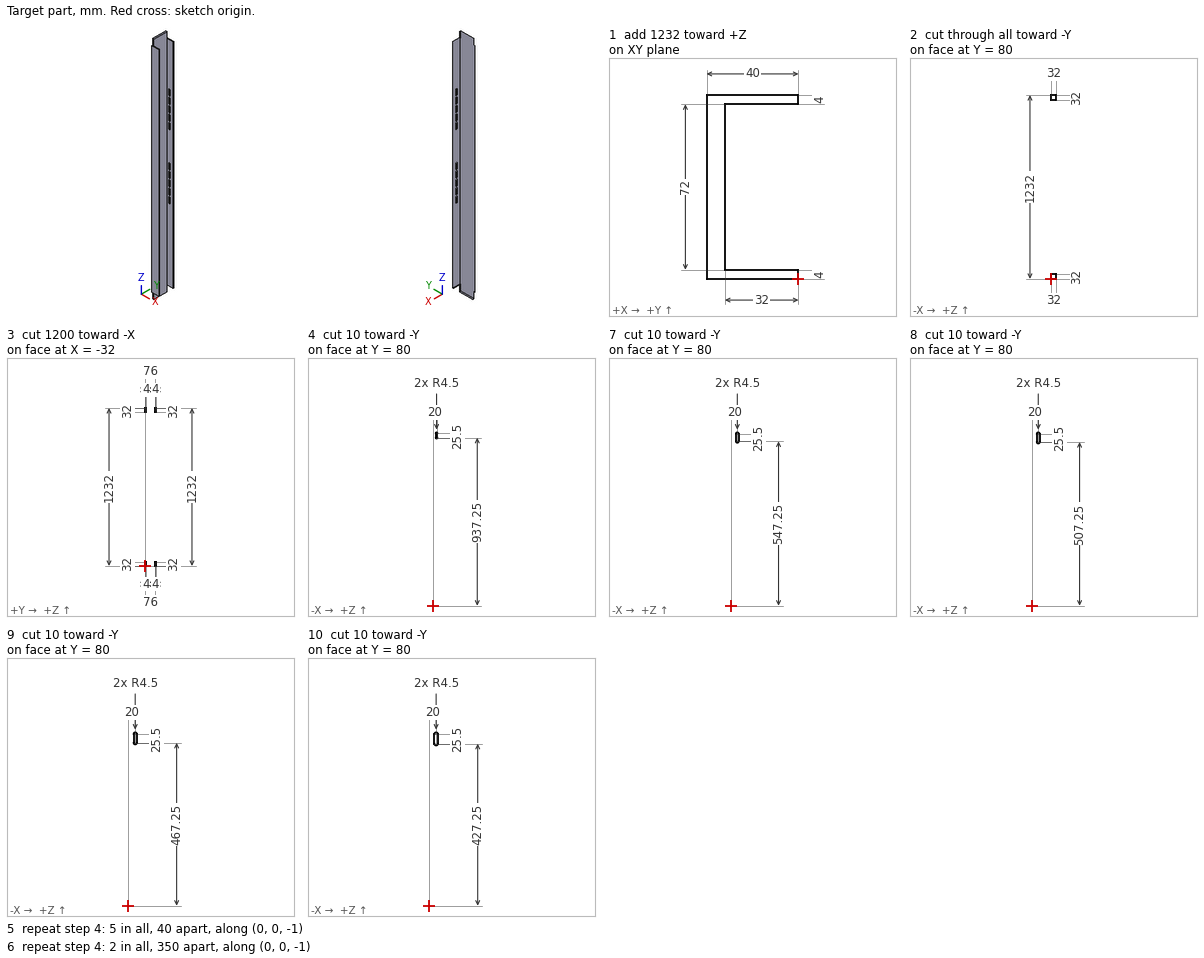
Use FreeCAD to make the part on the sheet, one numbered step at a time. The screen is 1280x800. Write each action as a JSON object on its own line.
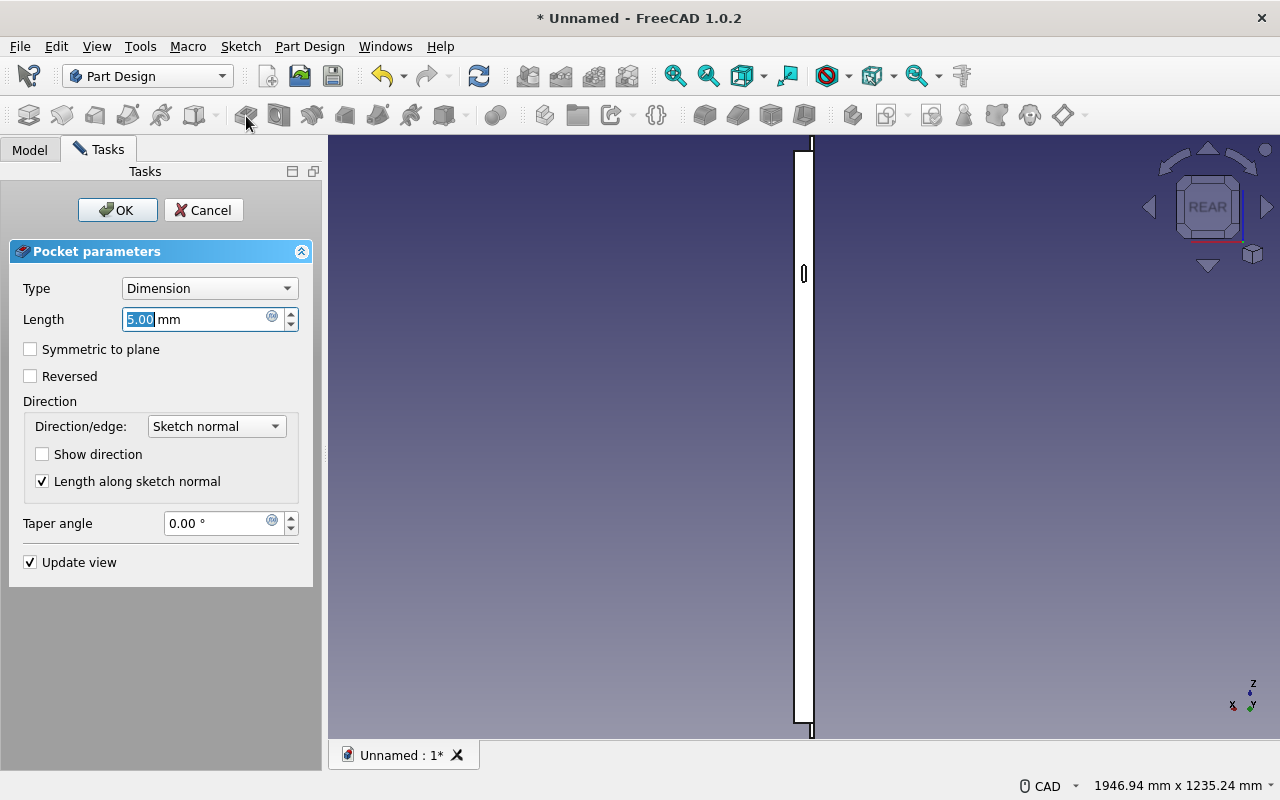
{"action": "type", "text": "10"}
{"action": "key", "text": "Tab"}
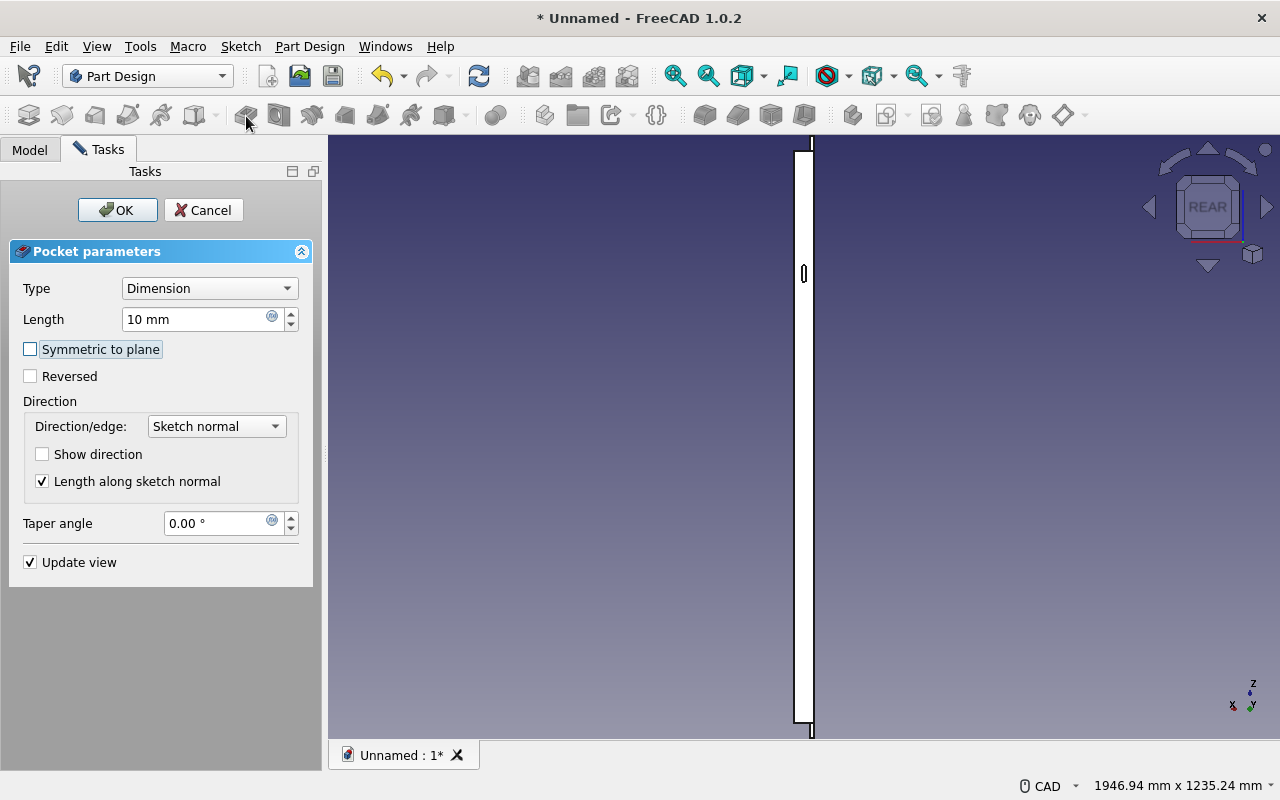
{"action": "left_click", "coordinate": [118, 210]}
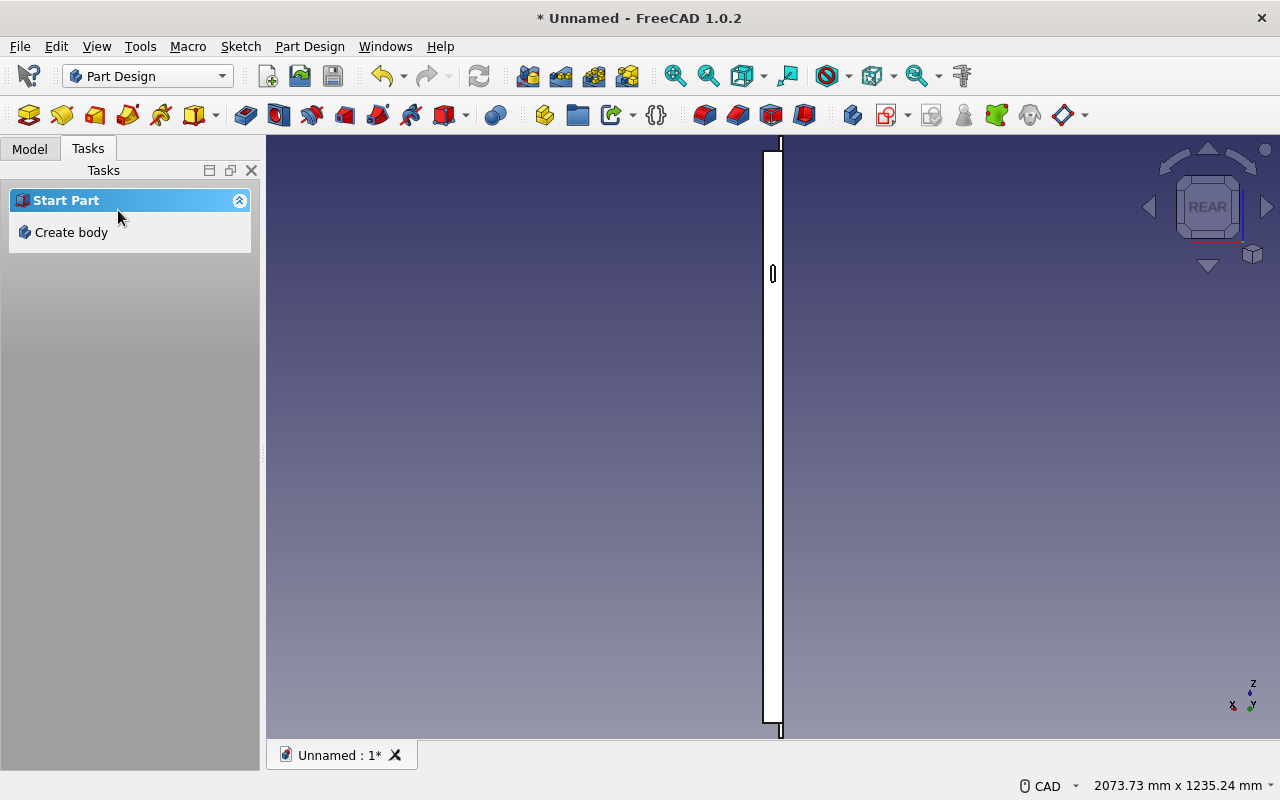
{"action": "left_click", "coordinate": [30, 148]}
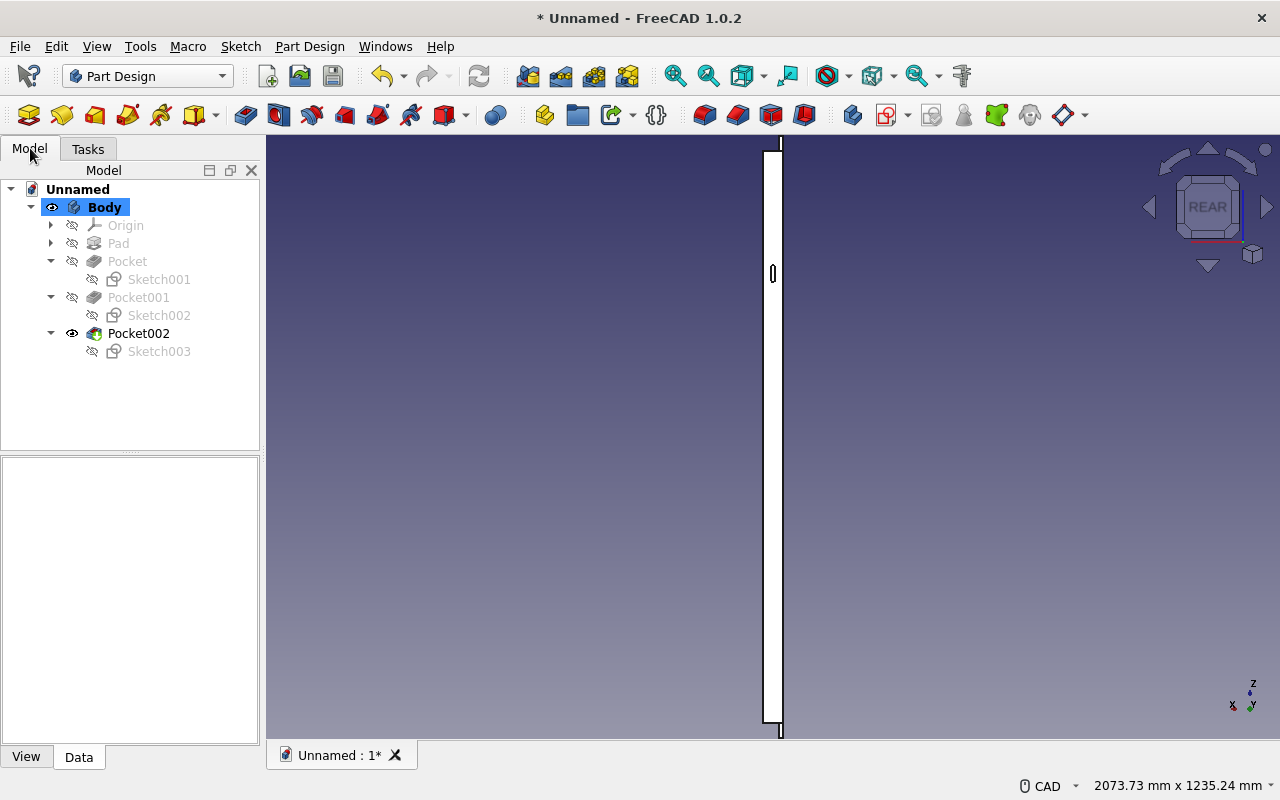
{"action": "left_click", "coordinate": [117, 333]}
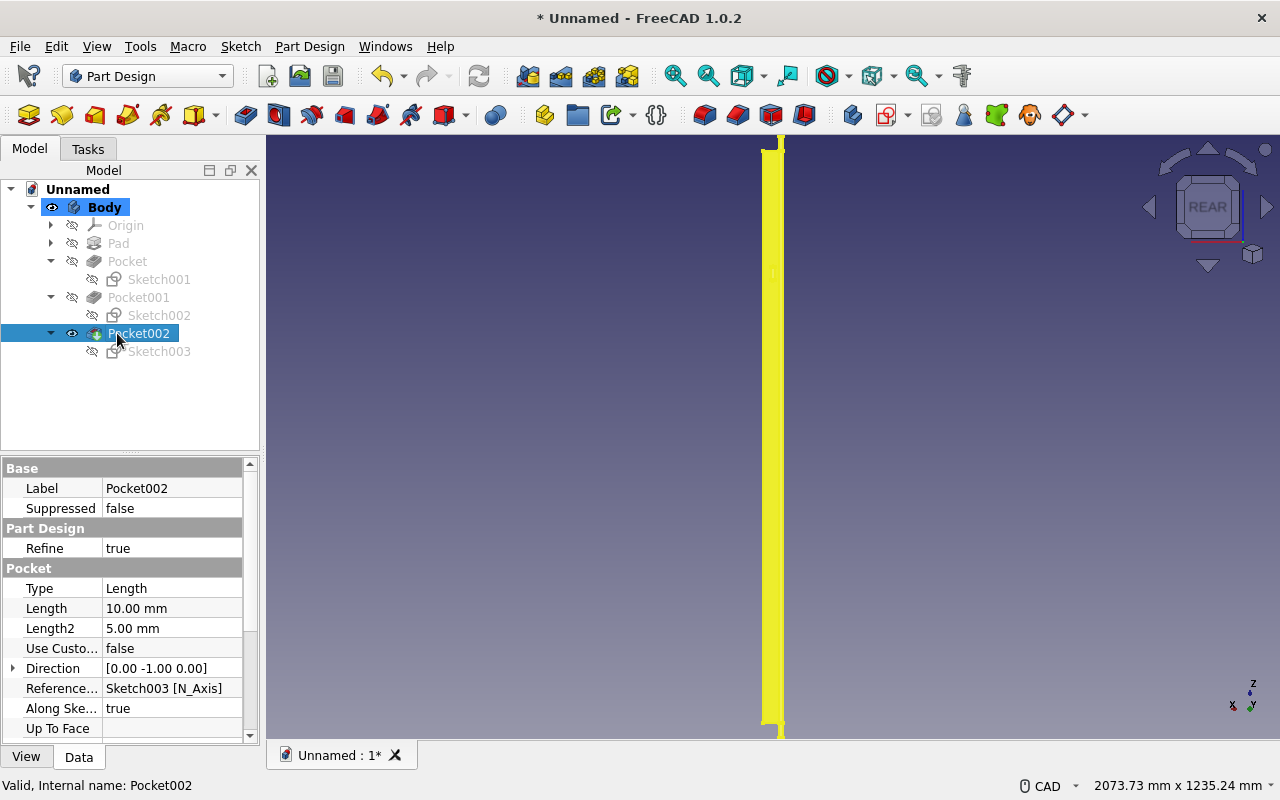
{"action": "left_click", "coordinate": [561, 76]}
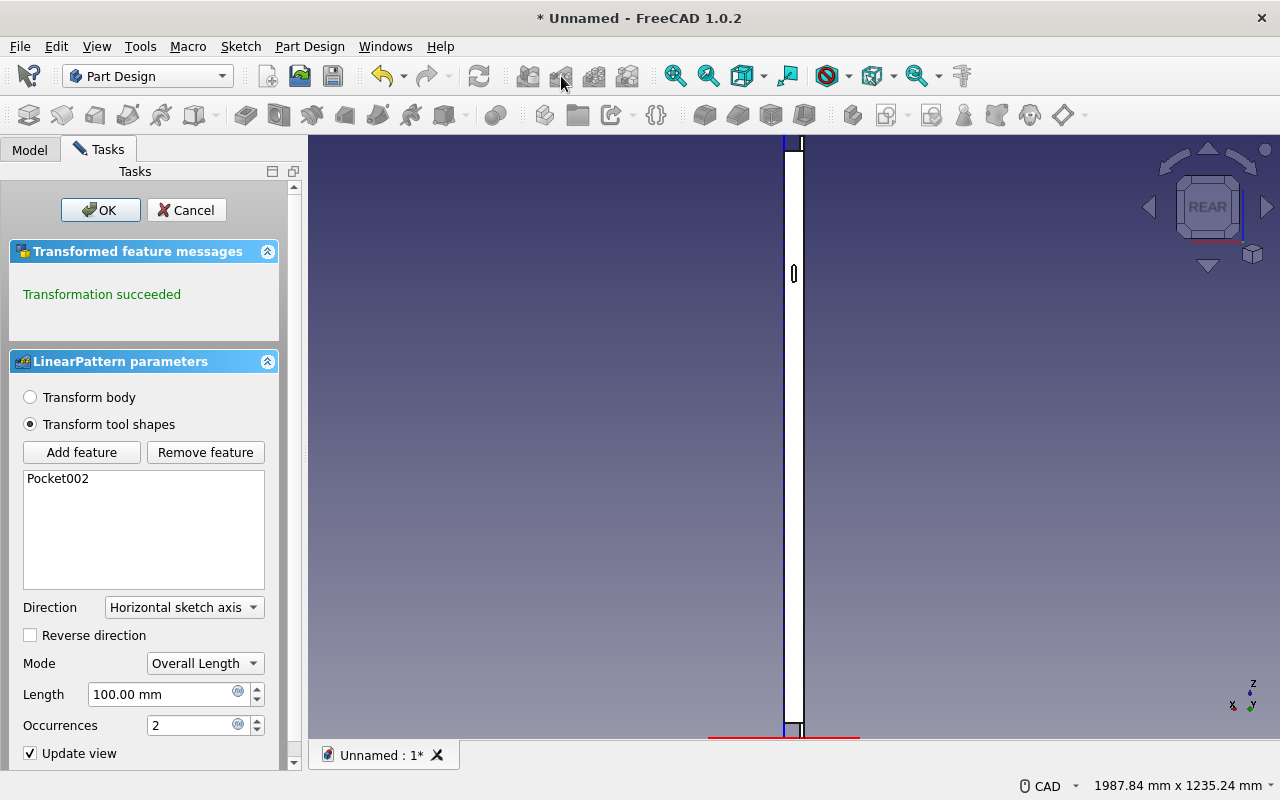
{"action": "left_click", "coordinate": [185, 608]}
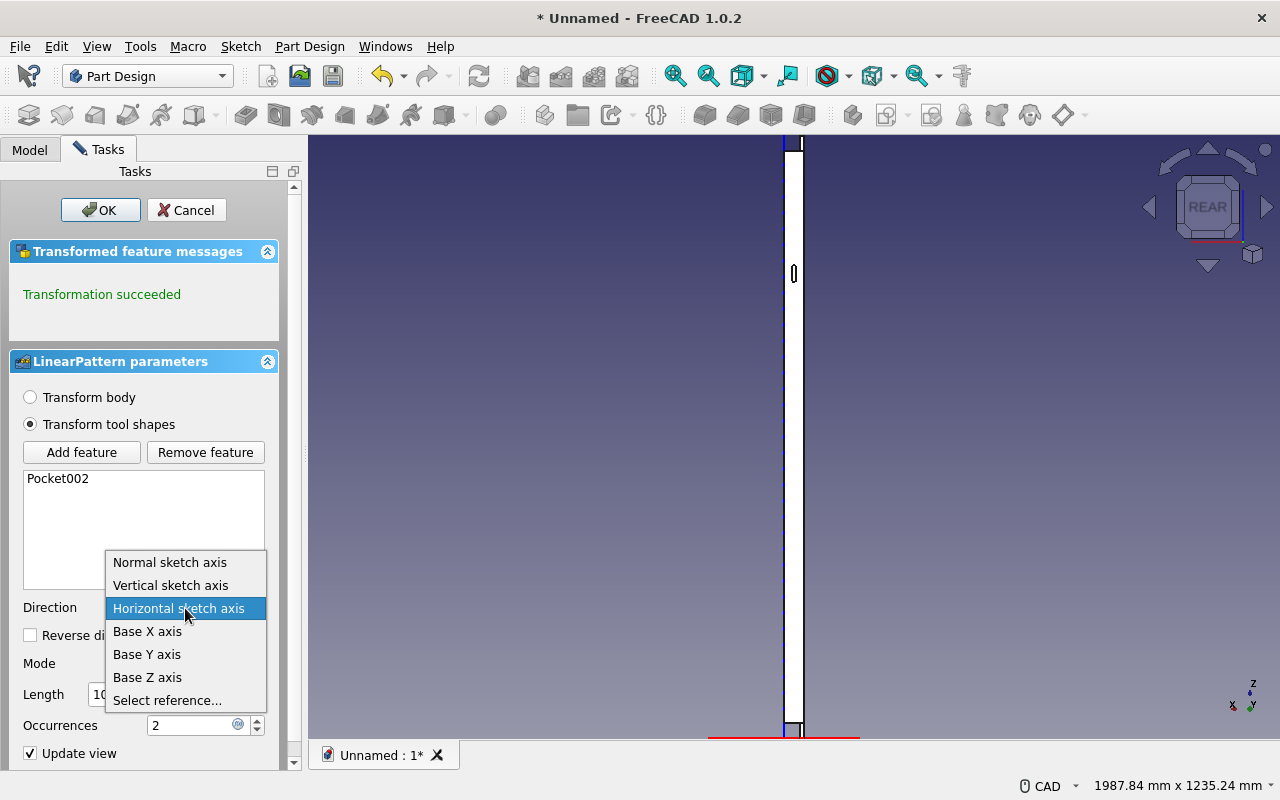
{"action": "left_click", "coordinate": [184, 678]}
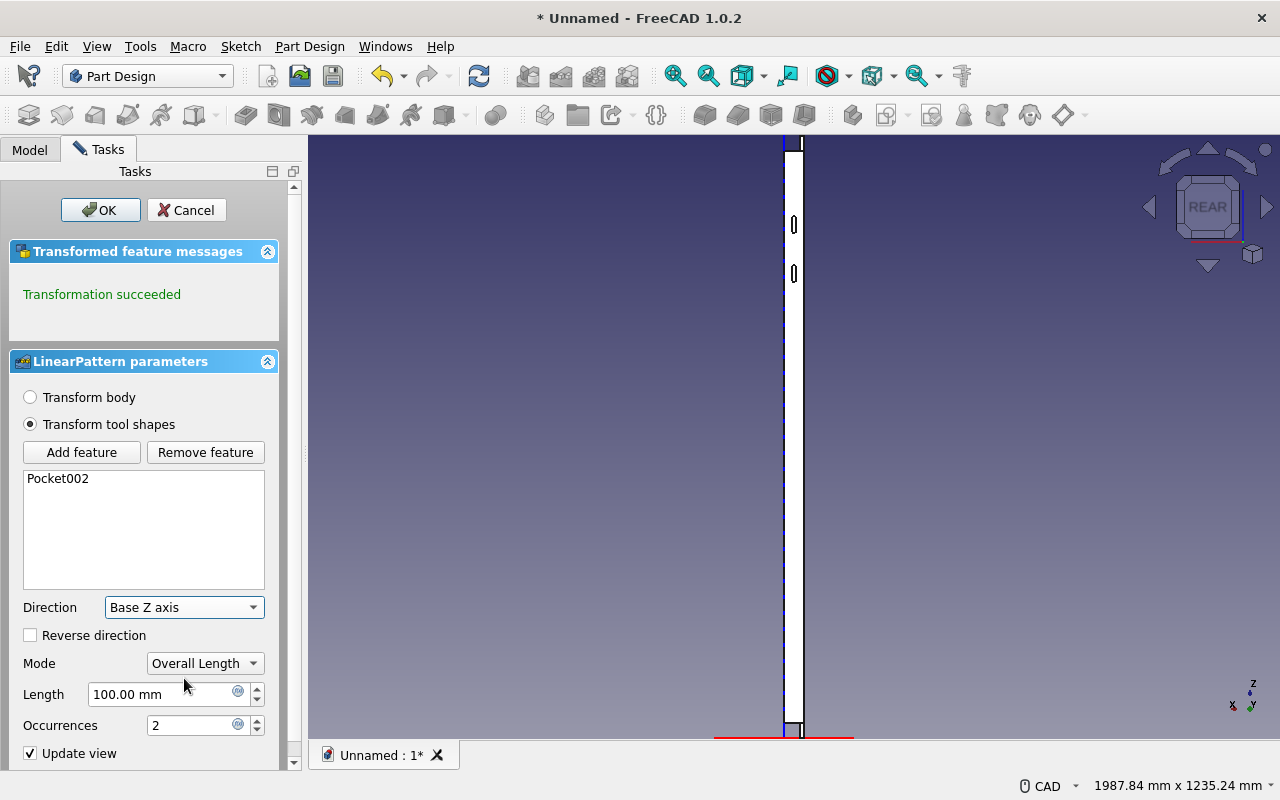
{"action": "left_click", "coordinate": [206, 664]}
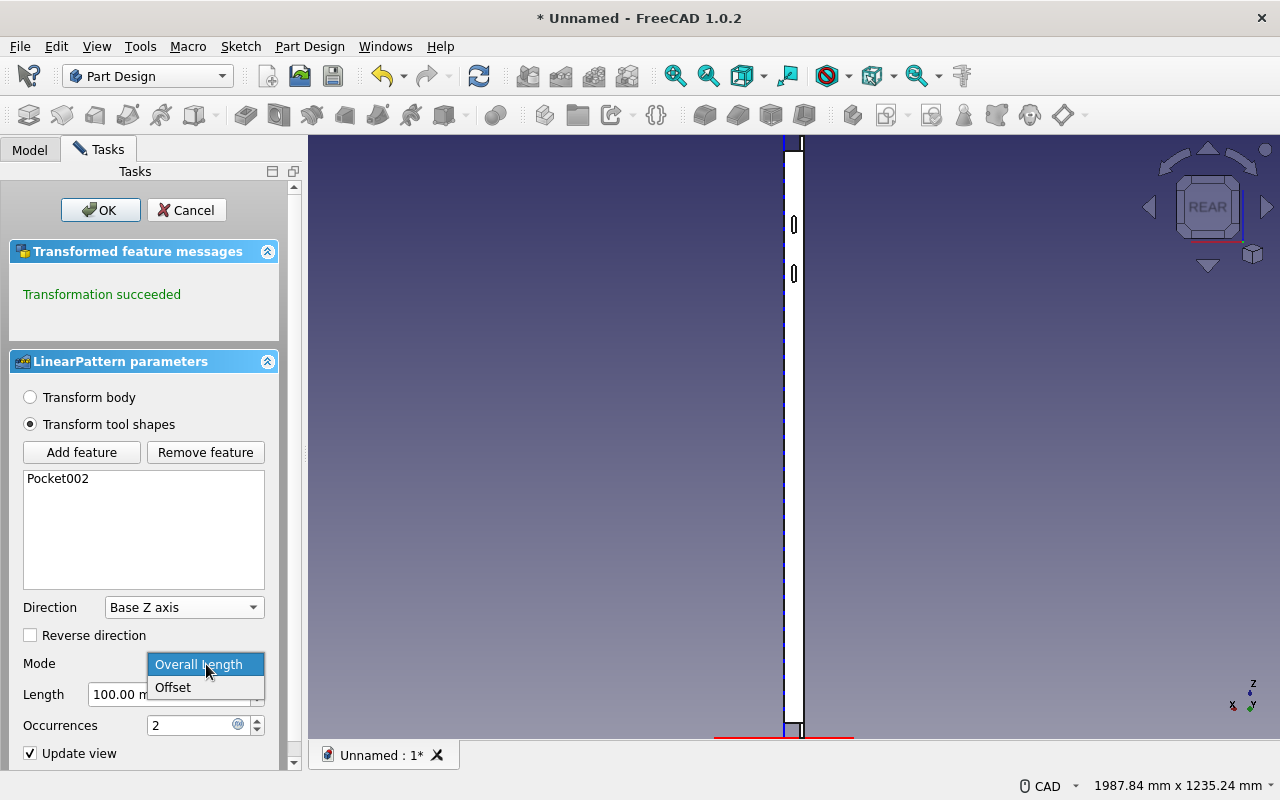
{"action": "left_click", "coordinate": [204, 688]}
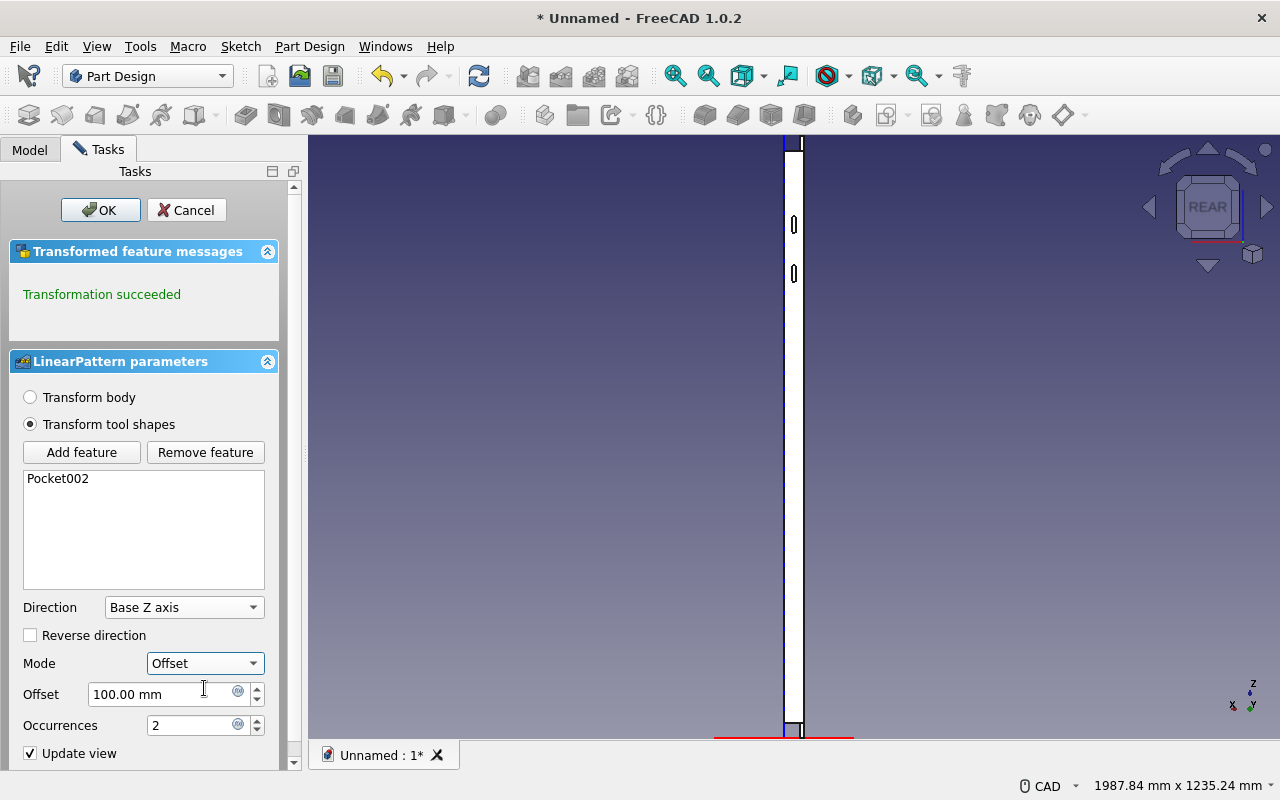
{"action": "triple_click", "coordinate": [170, 694]}